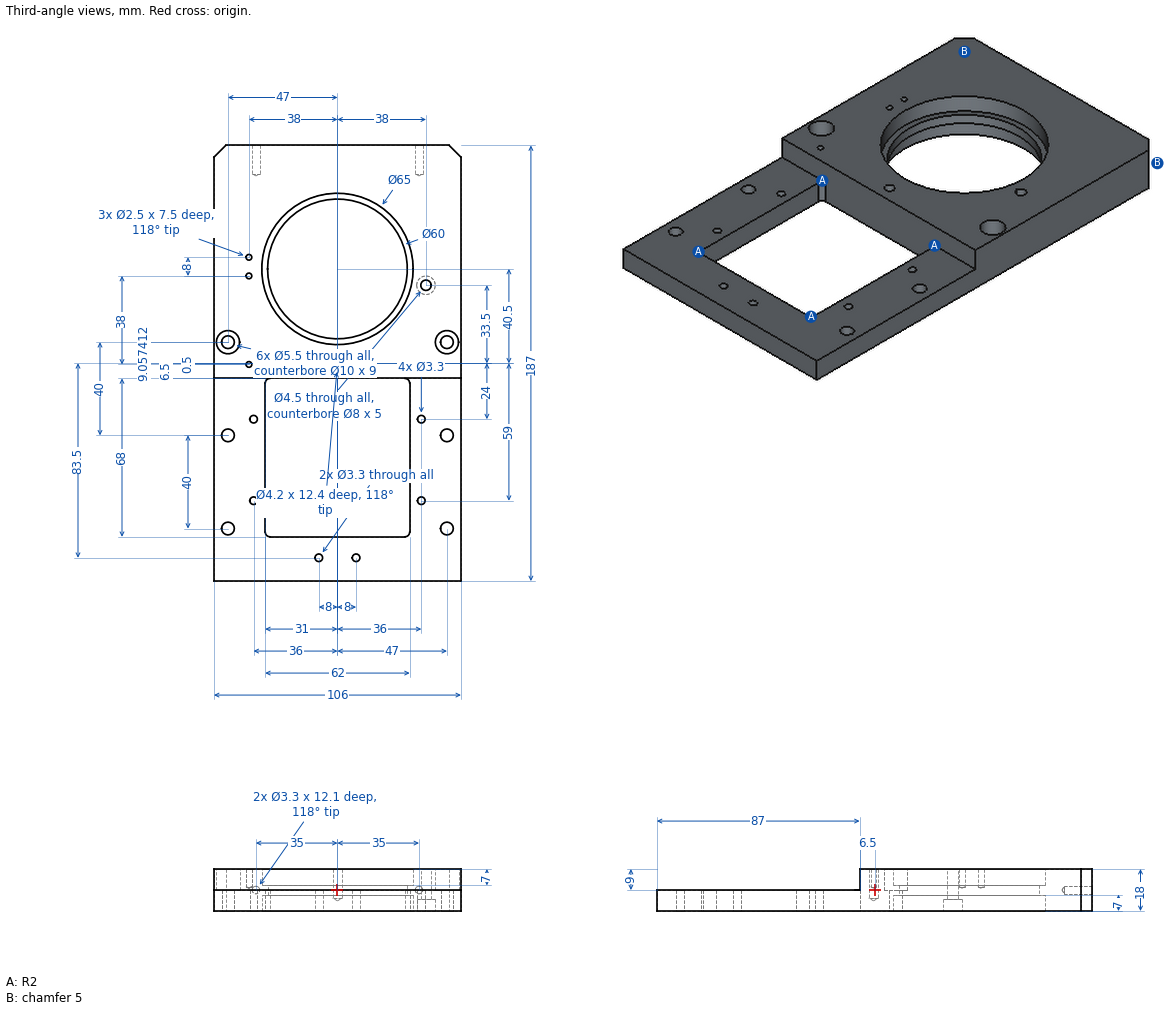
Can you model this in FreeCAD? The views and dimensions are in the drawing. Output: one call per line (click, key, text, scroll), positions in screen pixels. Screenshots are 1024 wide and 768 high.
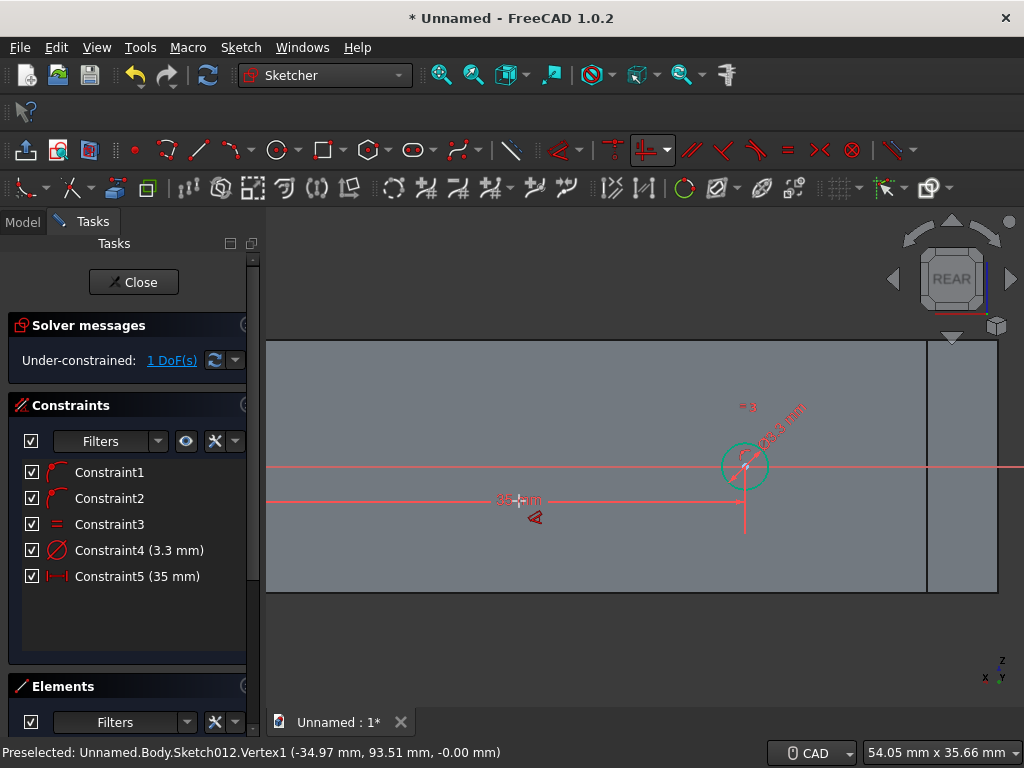
scroll(764, 451, down, 5)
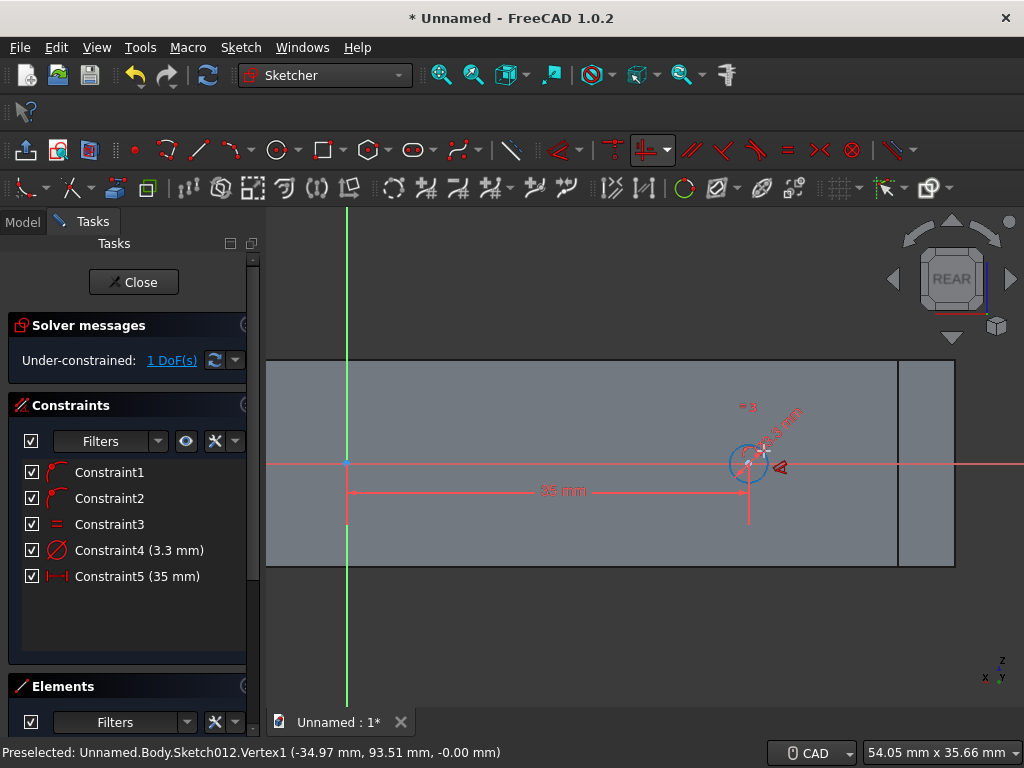
click(396, 457)
click(487, 491)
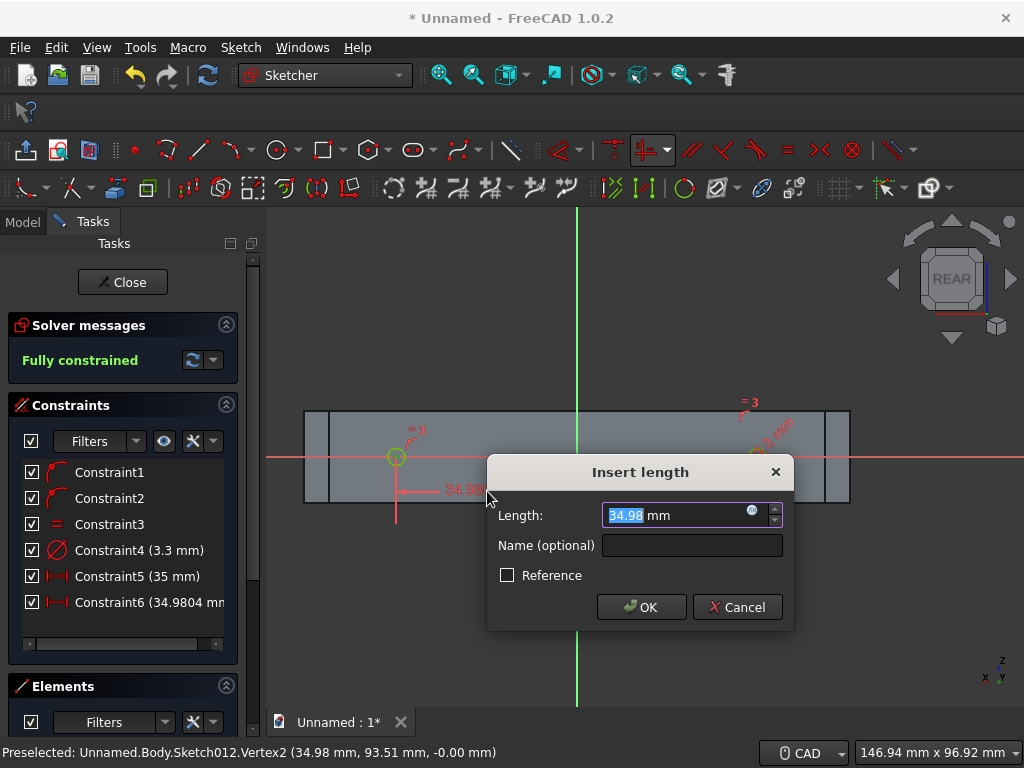
text(35)
key(Return)
key(Escape)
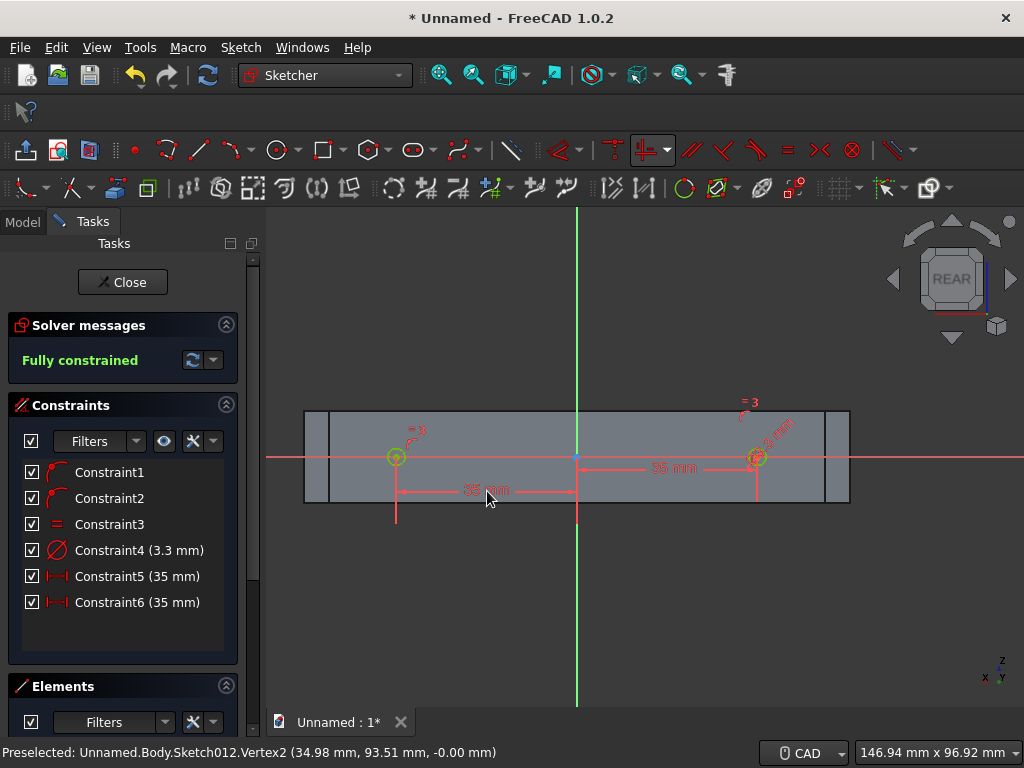
click(123, 282)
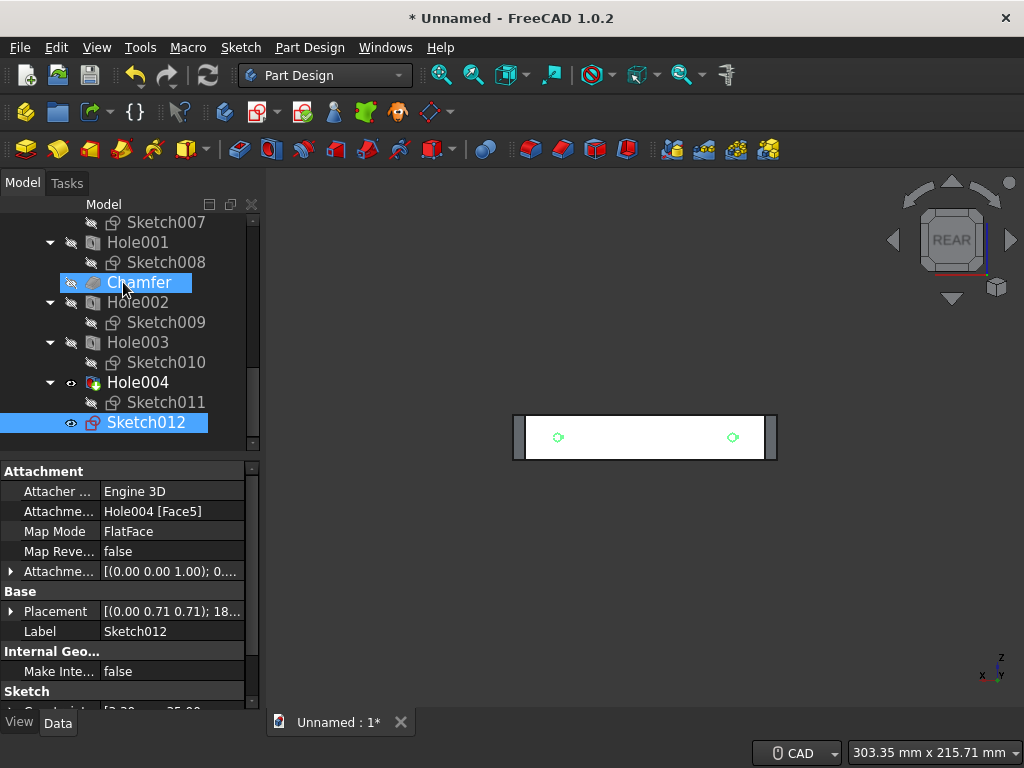
click(272, 150)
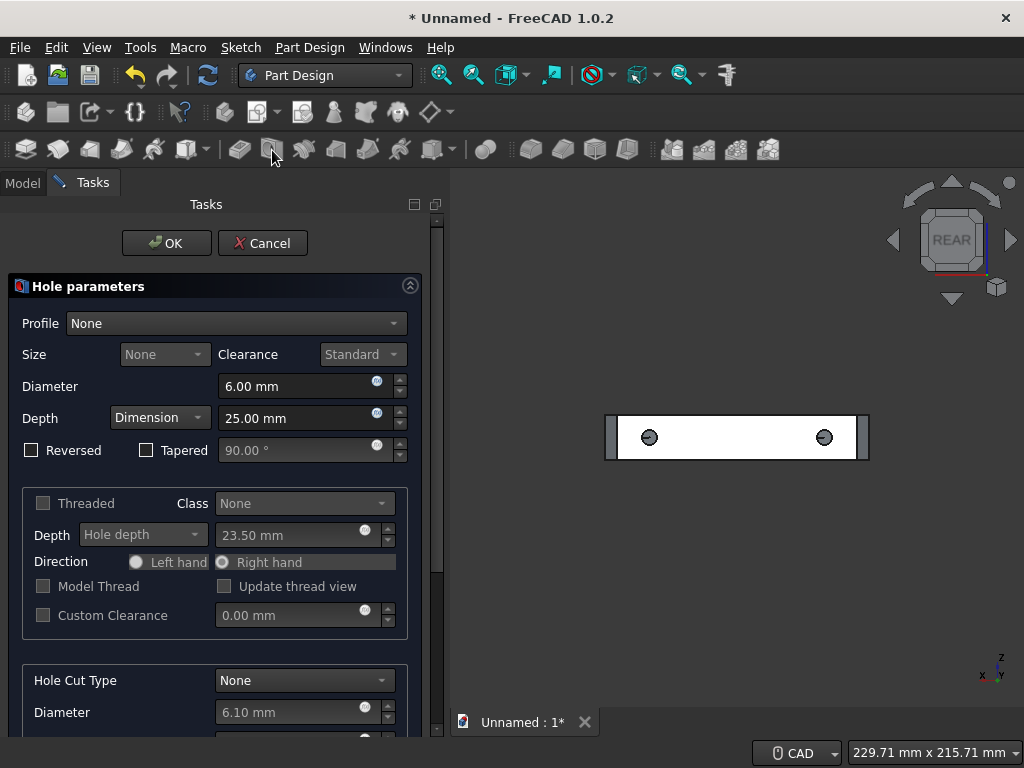
triple_click(305, 386)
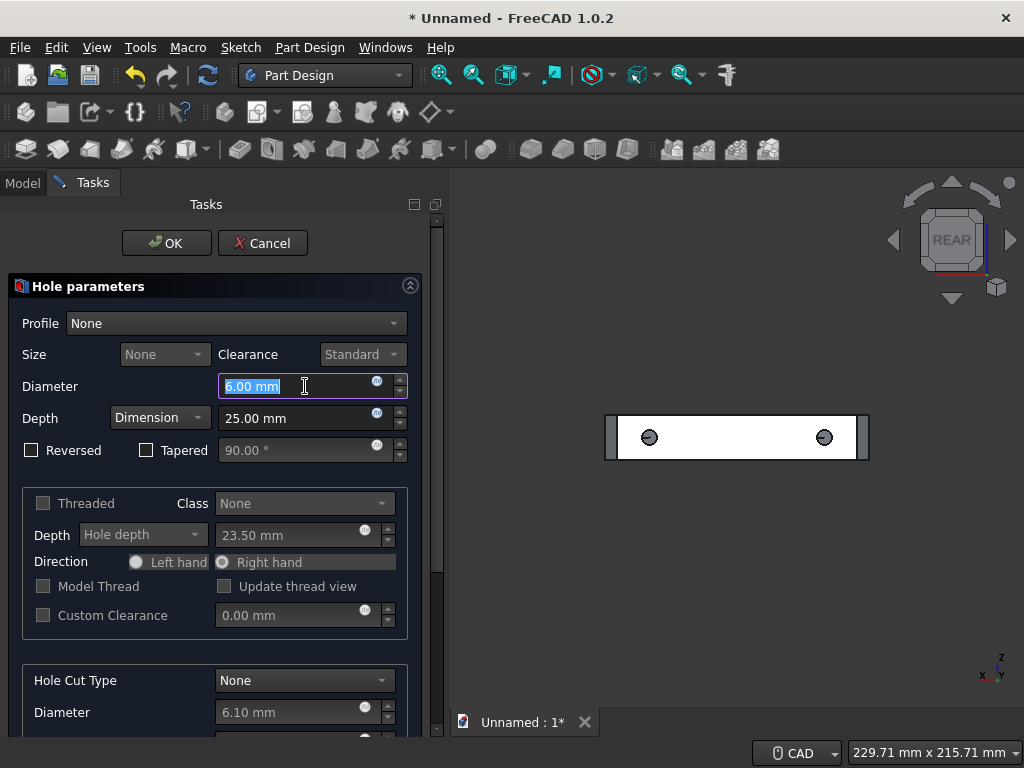
text(3.3)
key(Tab)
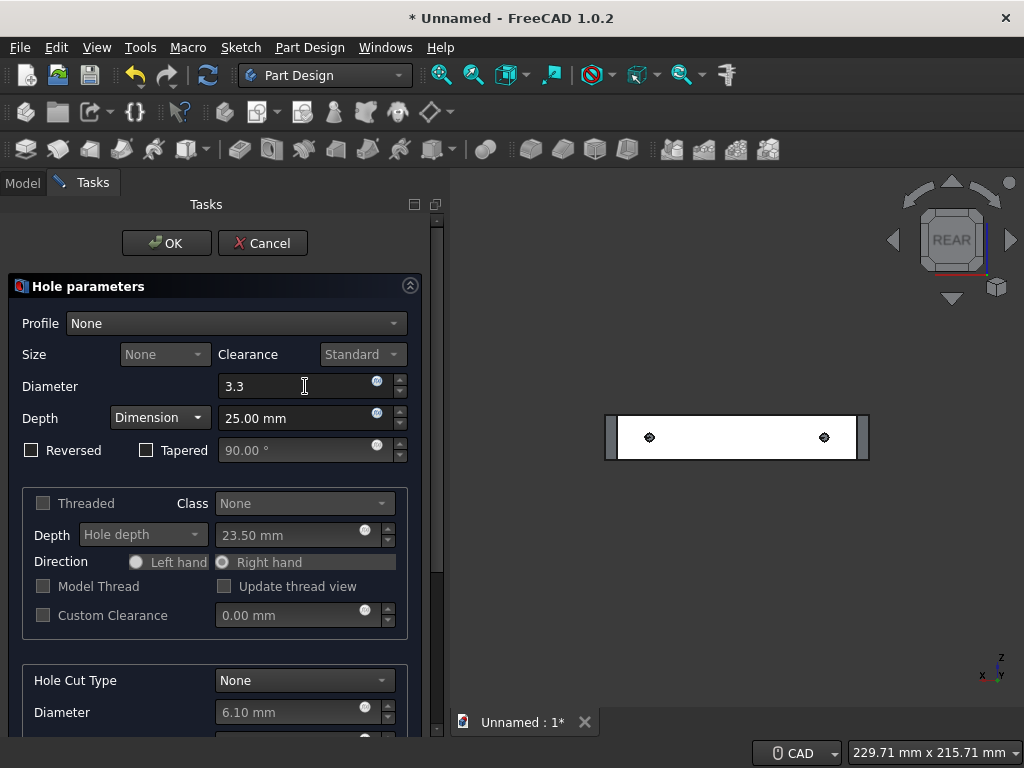
triple_click(305, 418)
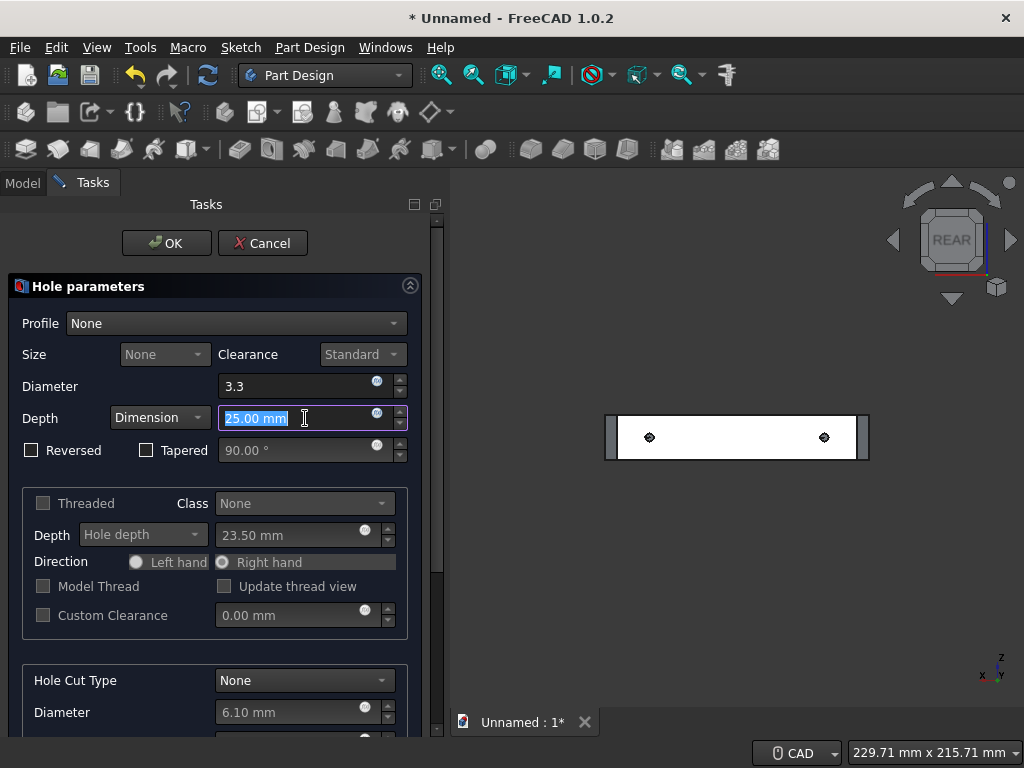
text(12.1)
key(Tab)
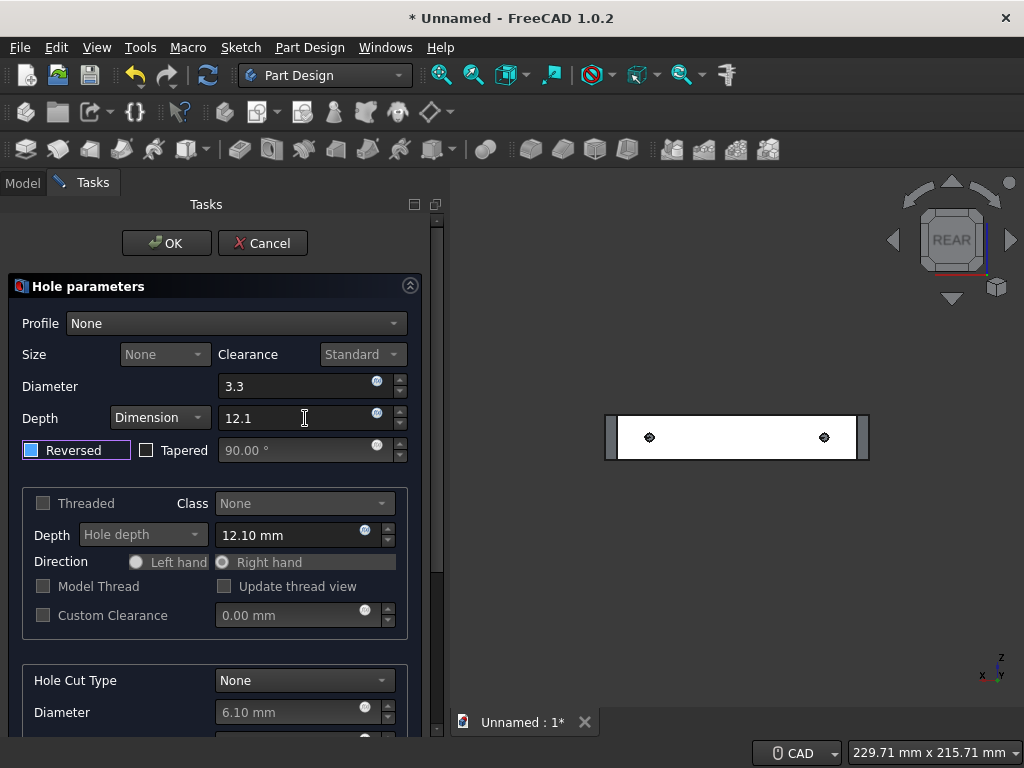
click(167, 243)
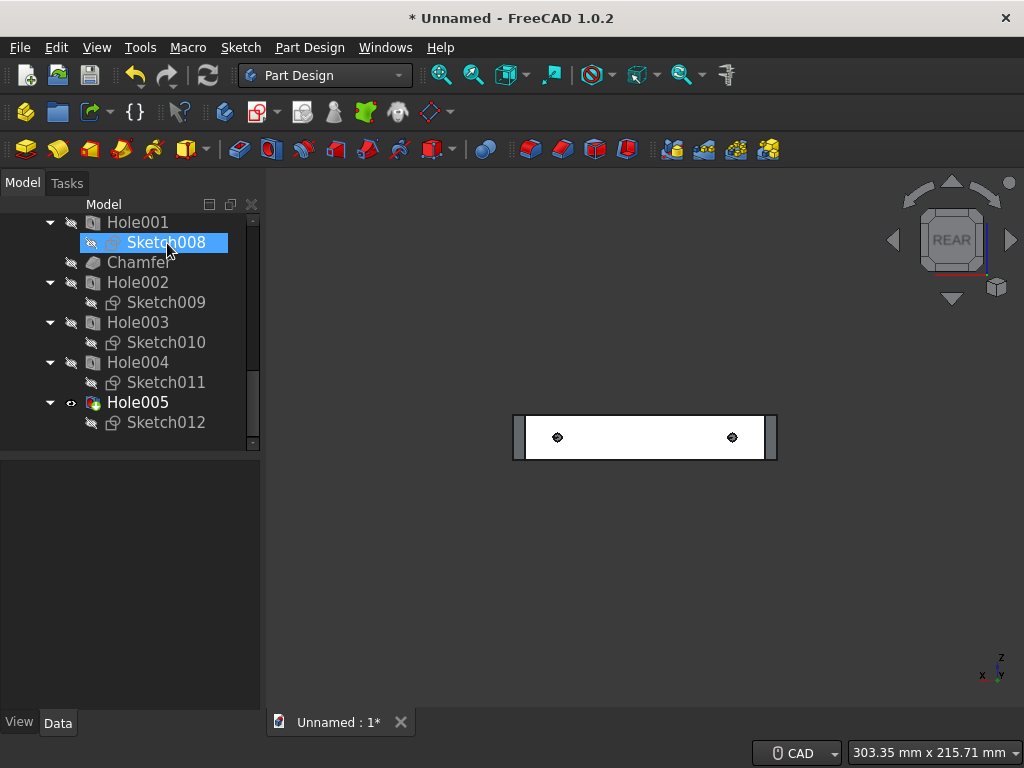
key(0)